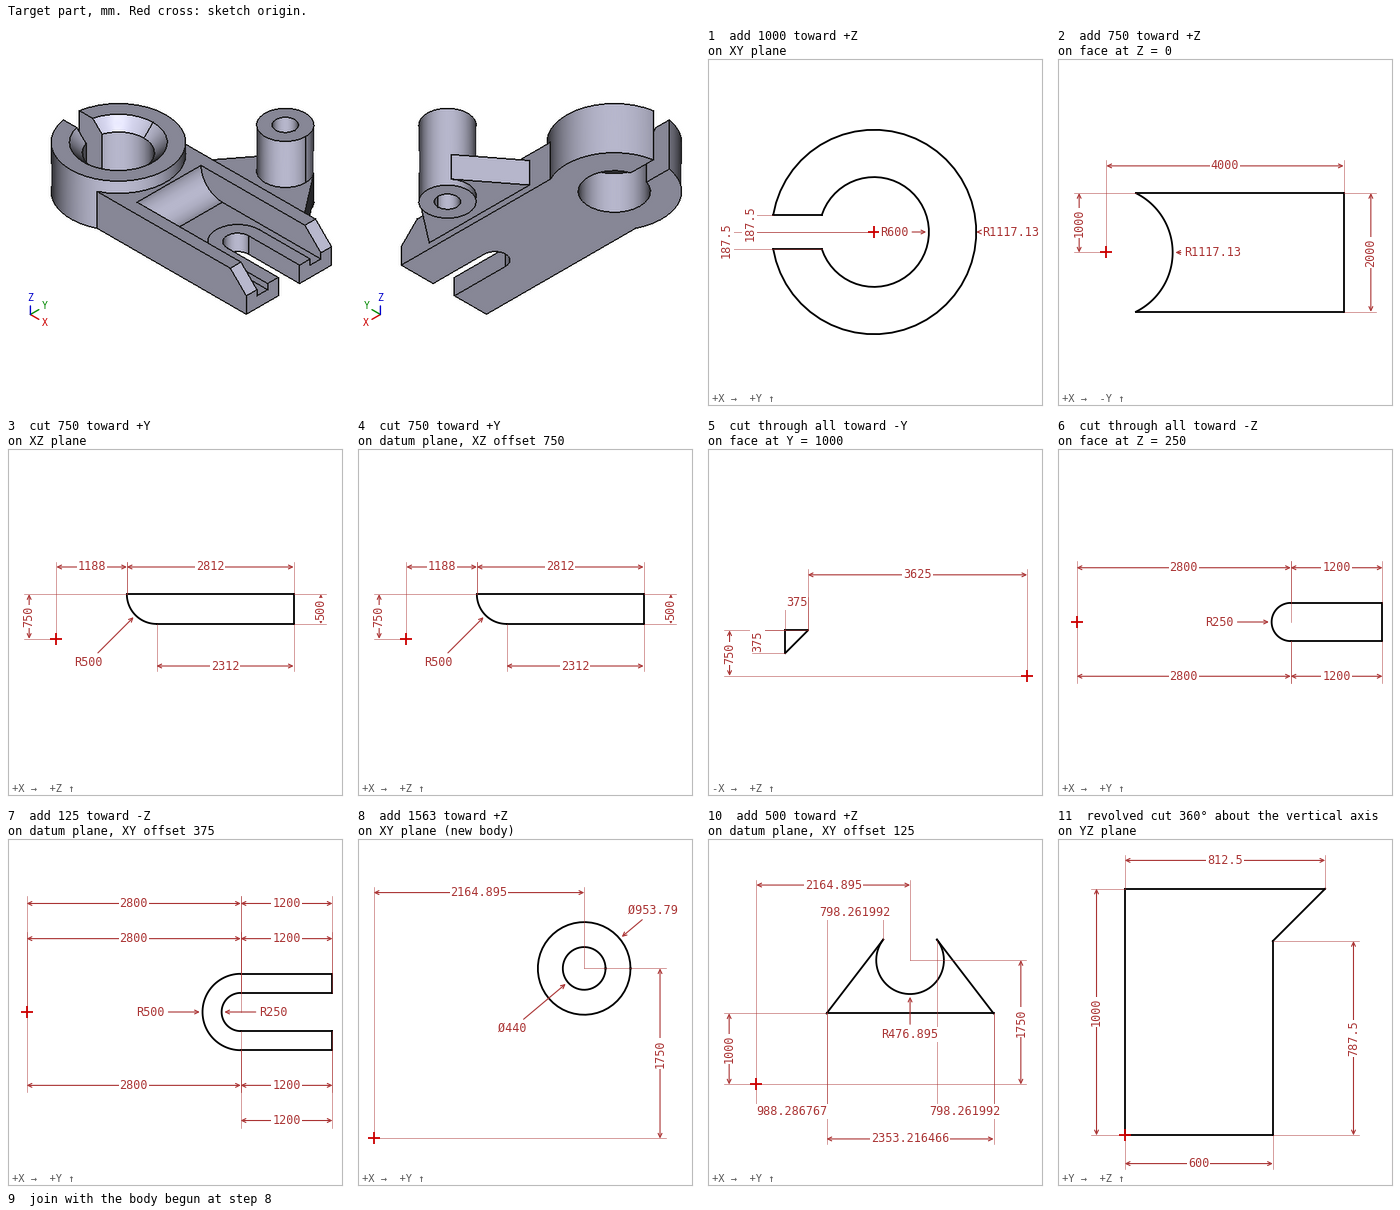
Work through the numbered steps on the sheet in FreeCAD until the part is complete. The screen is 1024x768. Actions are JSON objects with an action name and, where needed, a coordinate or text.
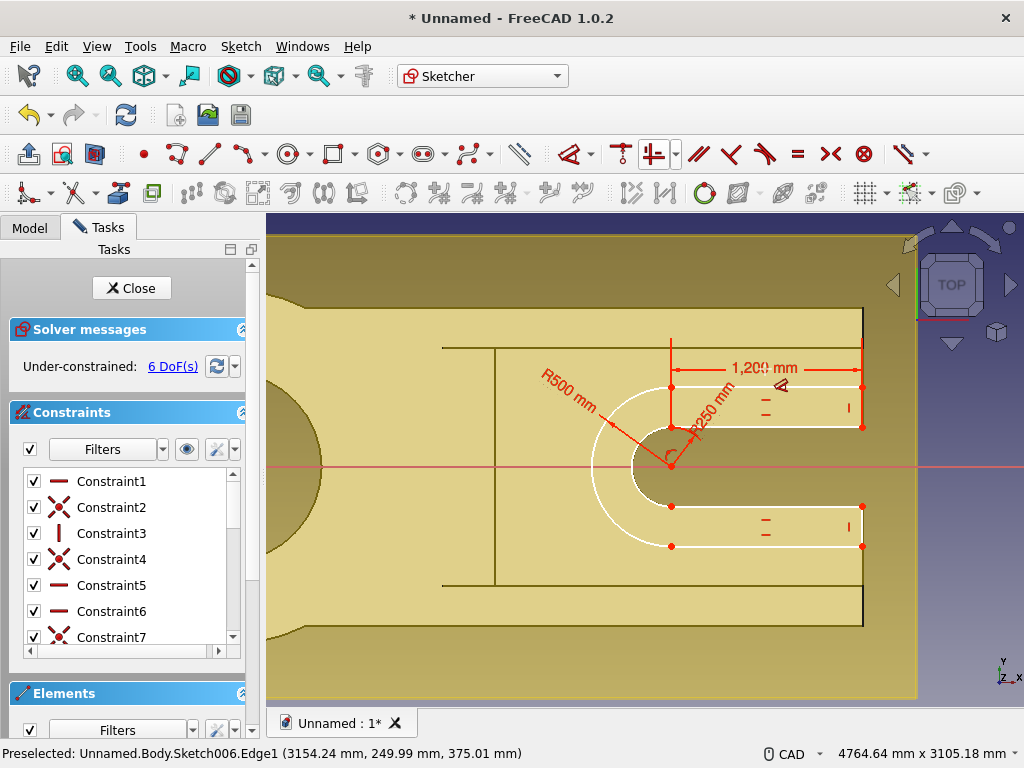
{"action": "left_click", "coordinate": [805, 387]}
{"action": "left_click", "coordinate": [765, 329]}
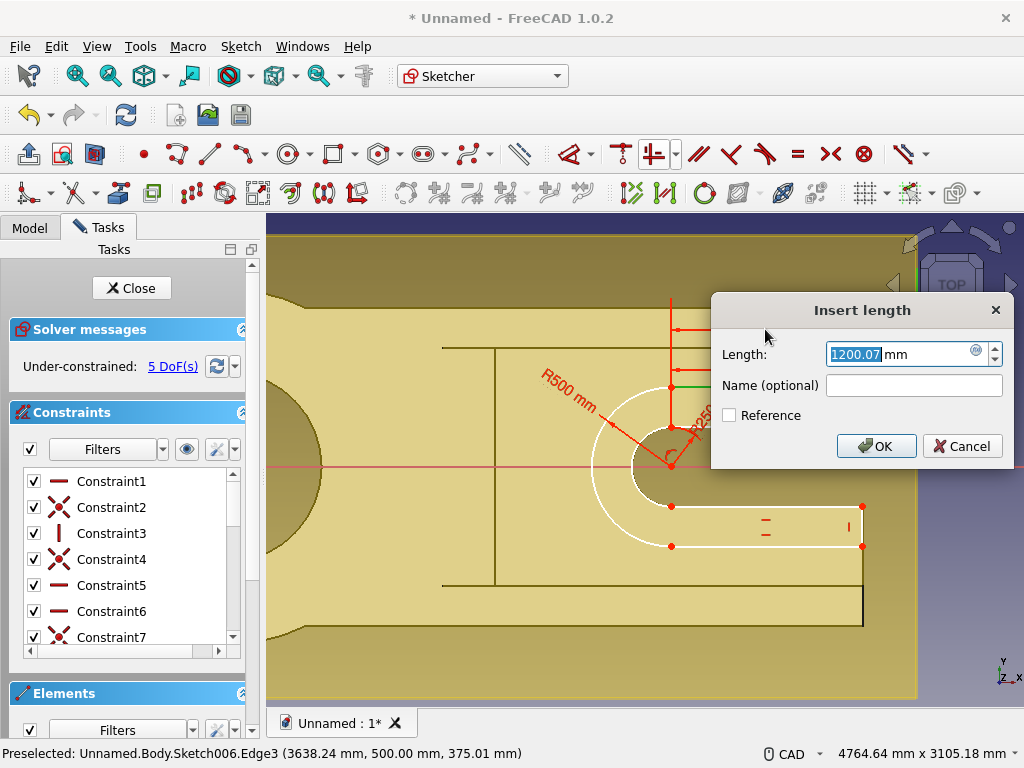
{"action": "type", "text": "1200"}
{"action": "key", "text": "Return"}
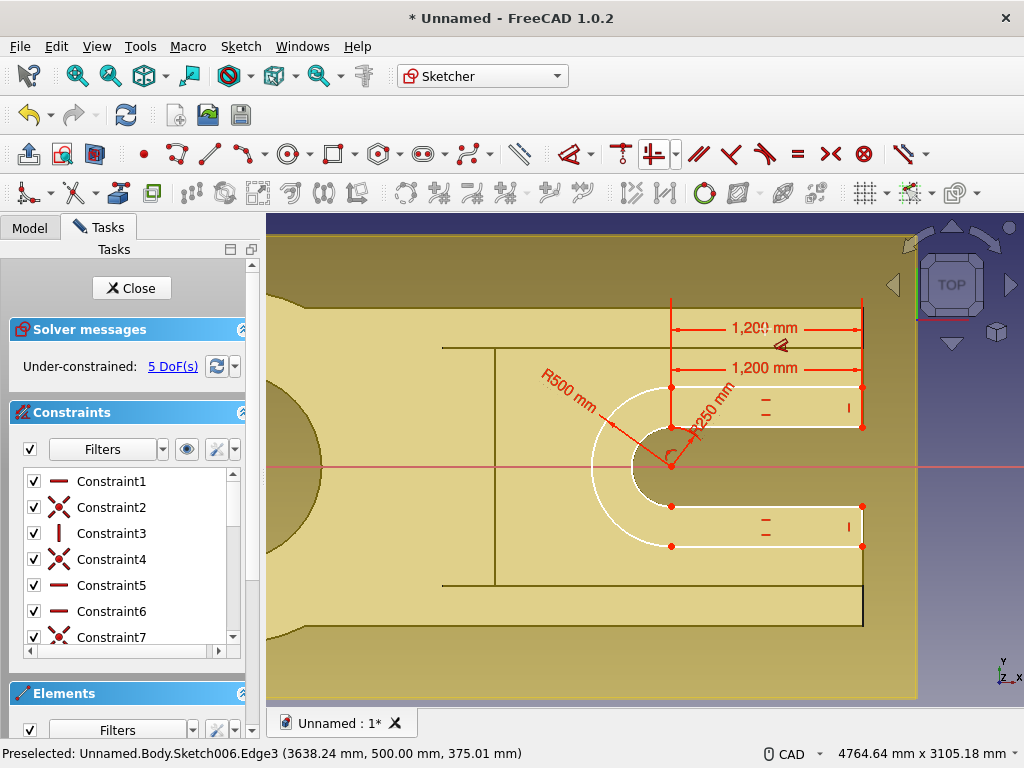
{"action": "left_click", "coordinate": [728, 547]}
{"action": "left_click", "coordinate": [765, 581]}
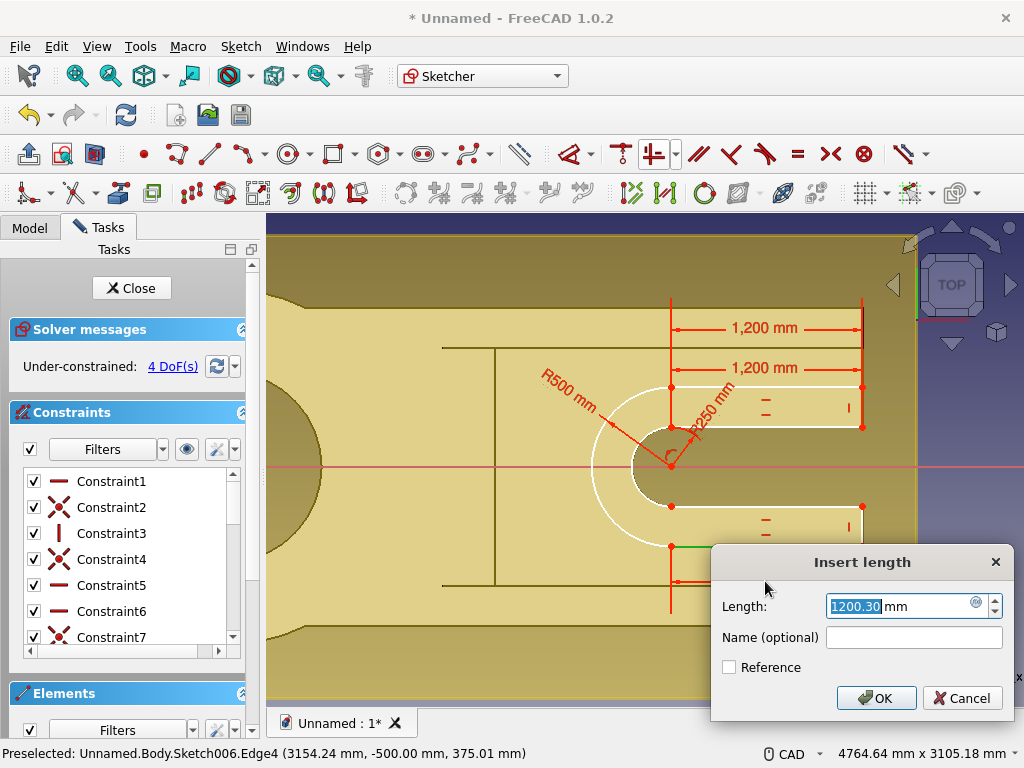
{"action": "type", "text": "1200"}
{"action": "key", "text": "Return"}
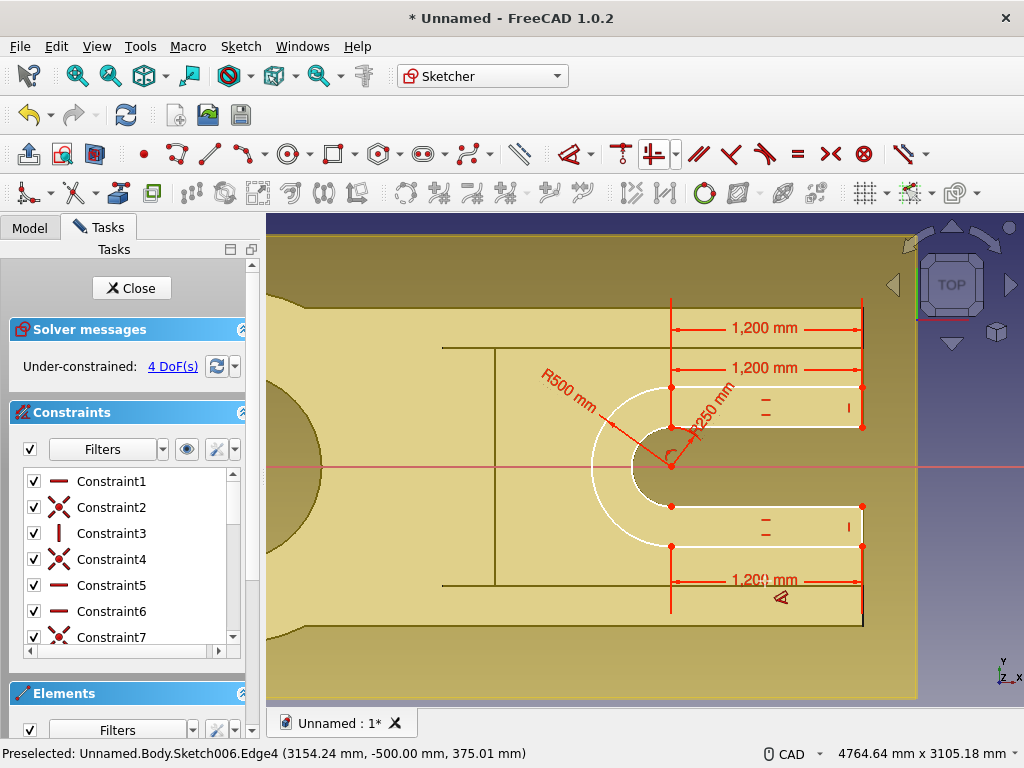
{"action": "left_click", "coordinate": [805, 507]}
{"action": "left_click", "coordinate": [765, 449]}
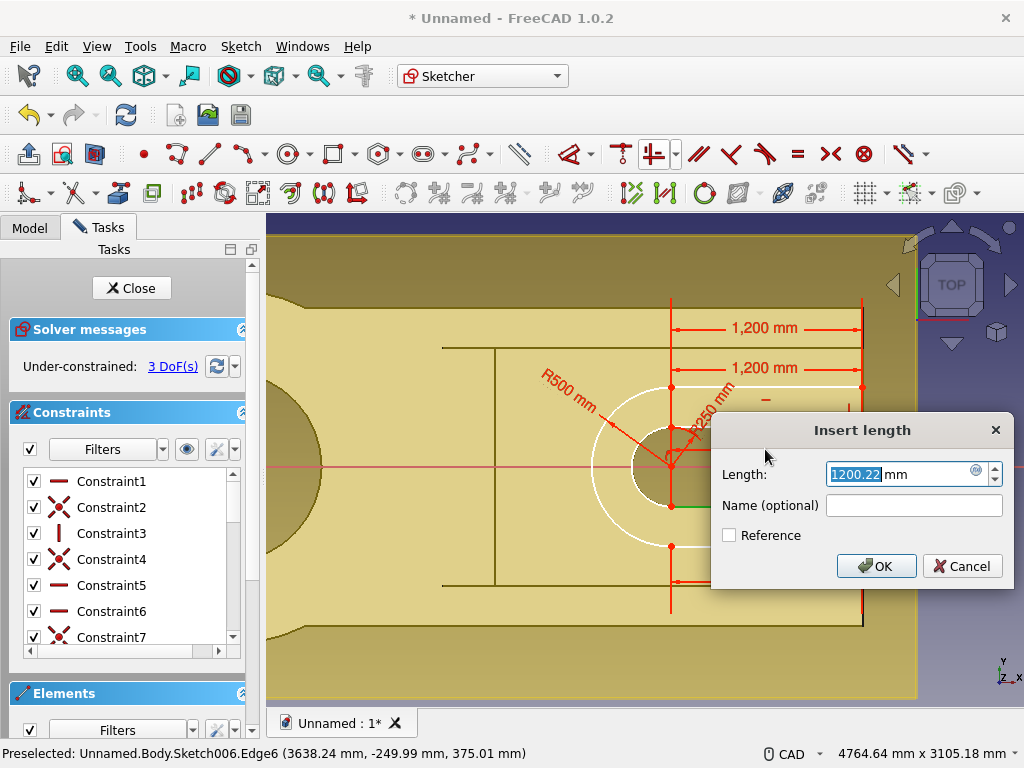
{"action": "type", "text": "1200"}
{"action": "key", "text": "Return"}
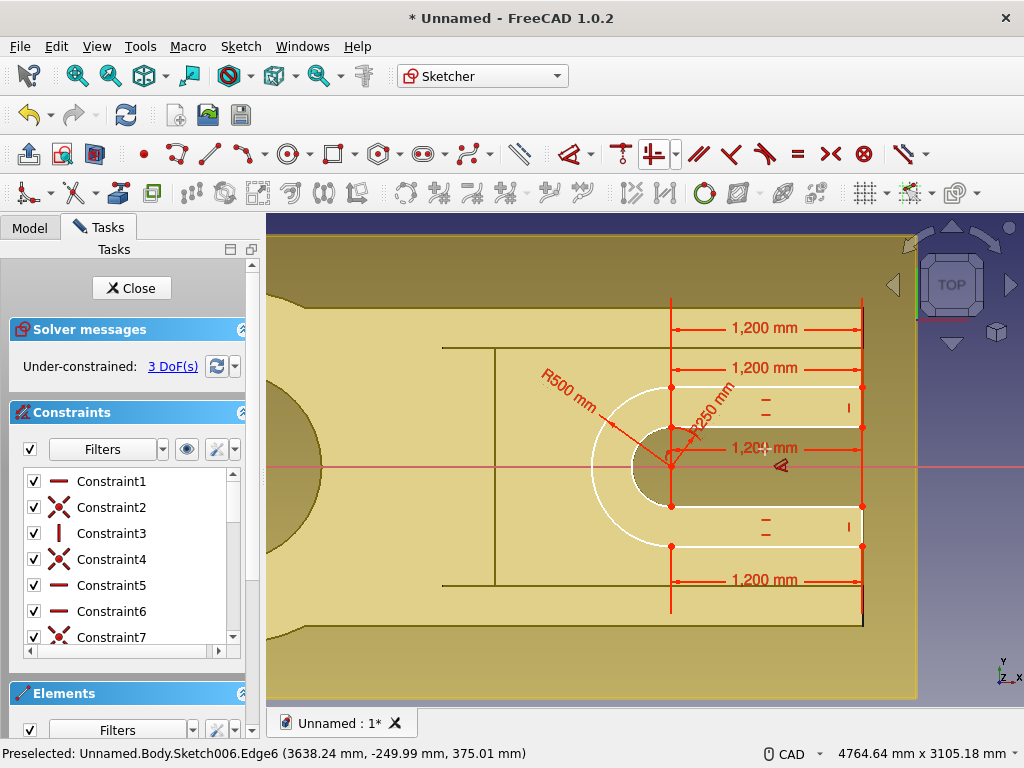
{"action": "left_click", "coordinate": [671, 427]}
{"action": "left_click", "coordinate": [483, 393]}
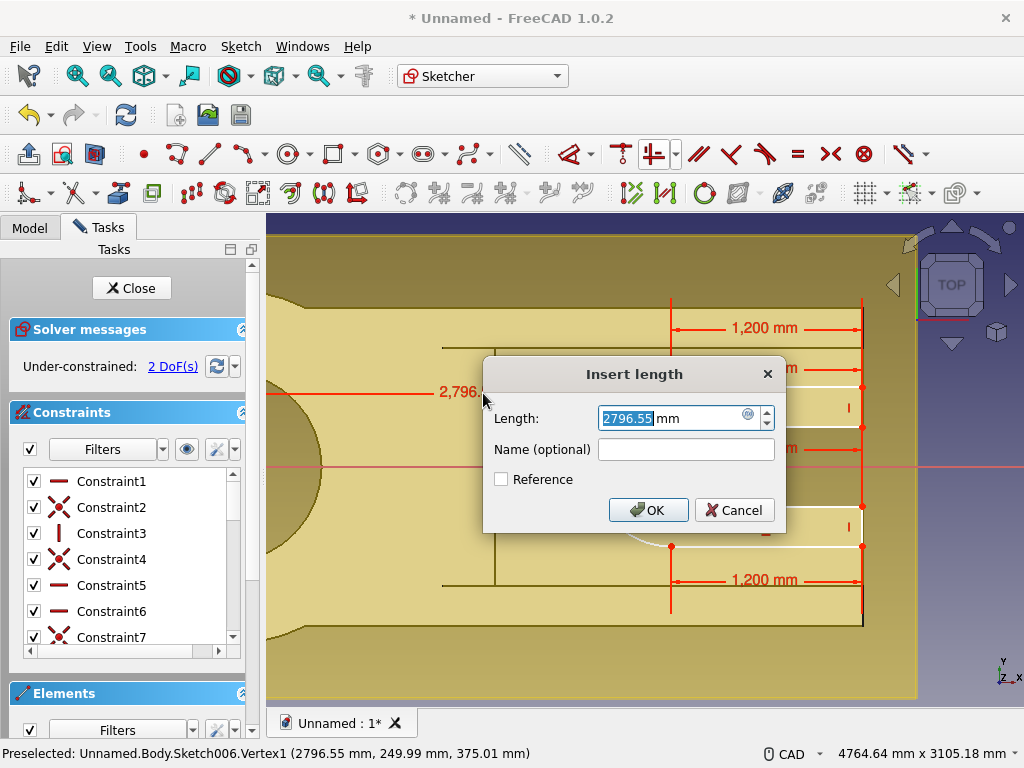
{"action": "type", "text": "2800"}
{"action": "key", "text": "Return"}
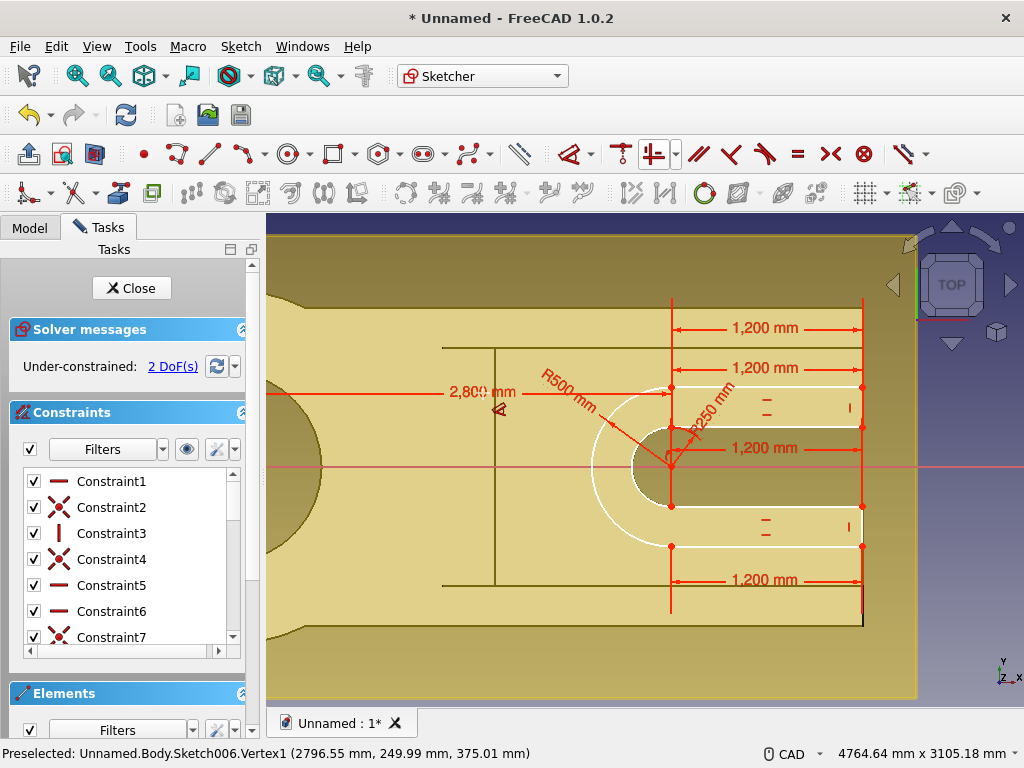
{"action": "left_click", "coordinate": [671, 547]}
{"action": "left_click", "coordinate": [483, 581]}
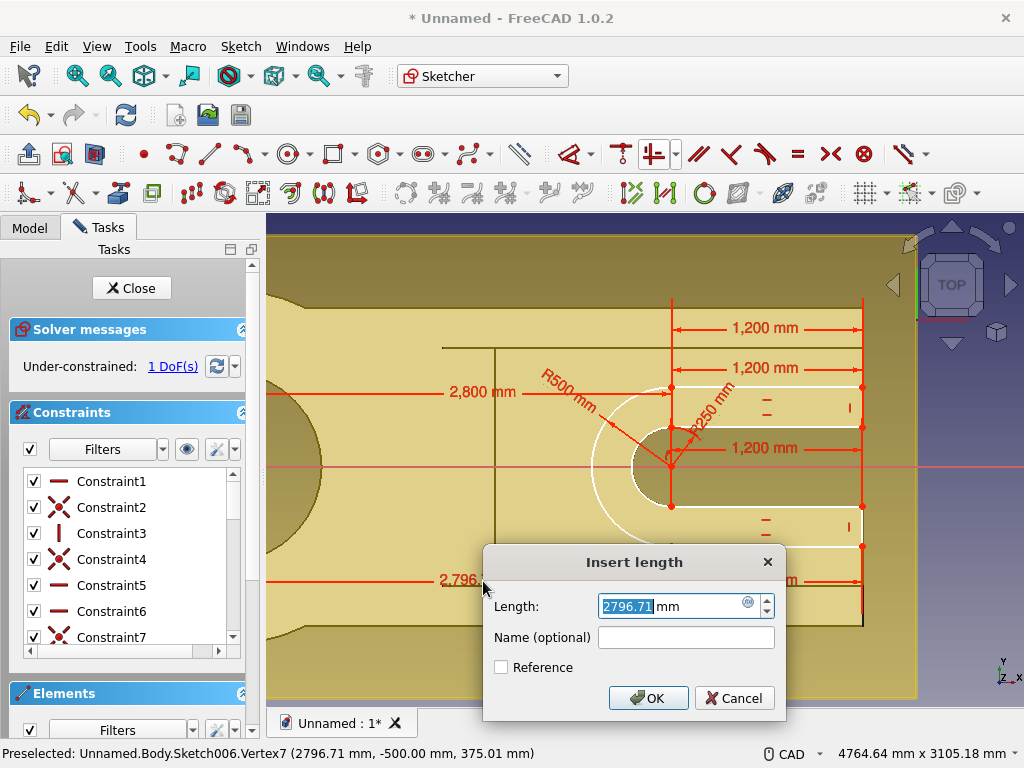
{"action": "type", "text": "2800"}
{"action": "key", "text": "Return"}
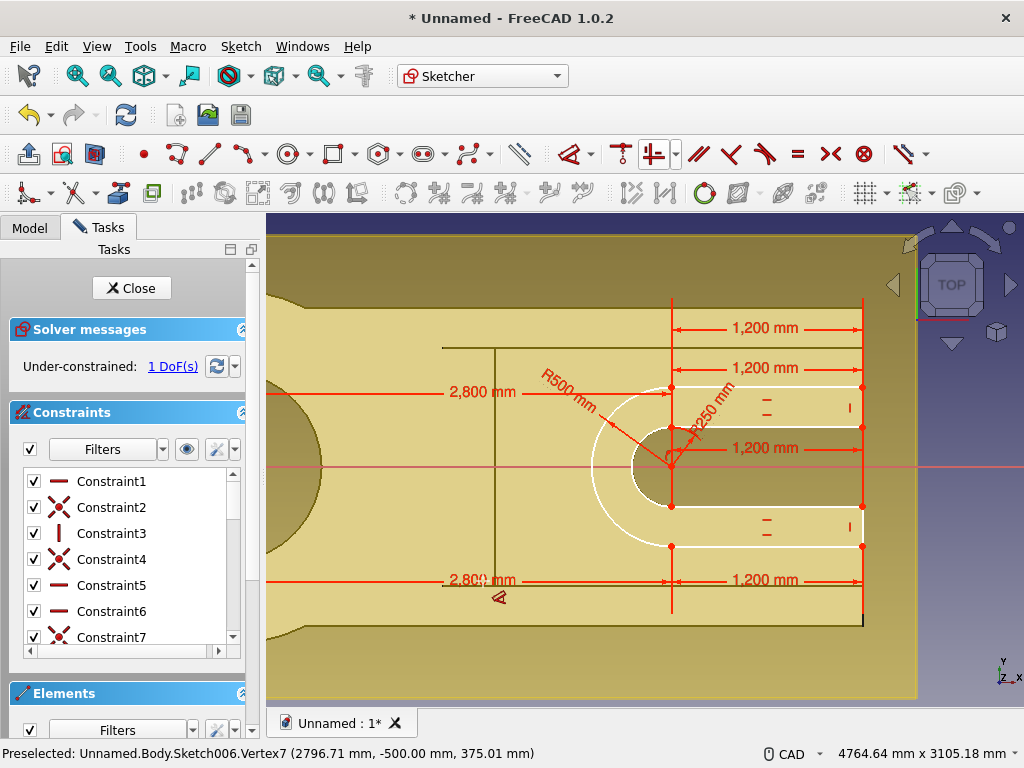
{"action": "left_click", "coordinate": [671, 467]}
{"action": "left_click", "coordinate": [483, 501]}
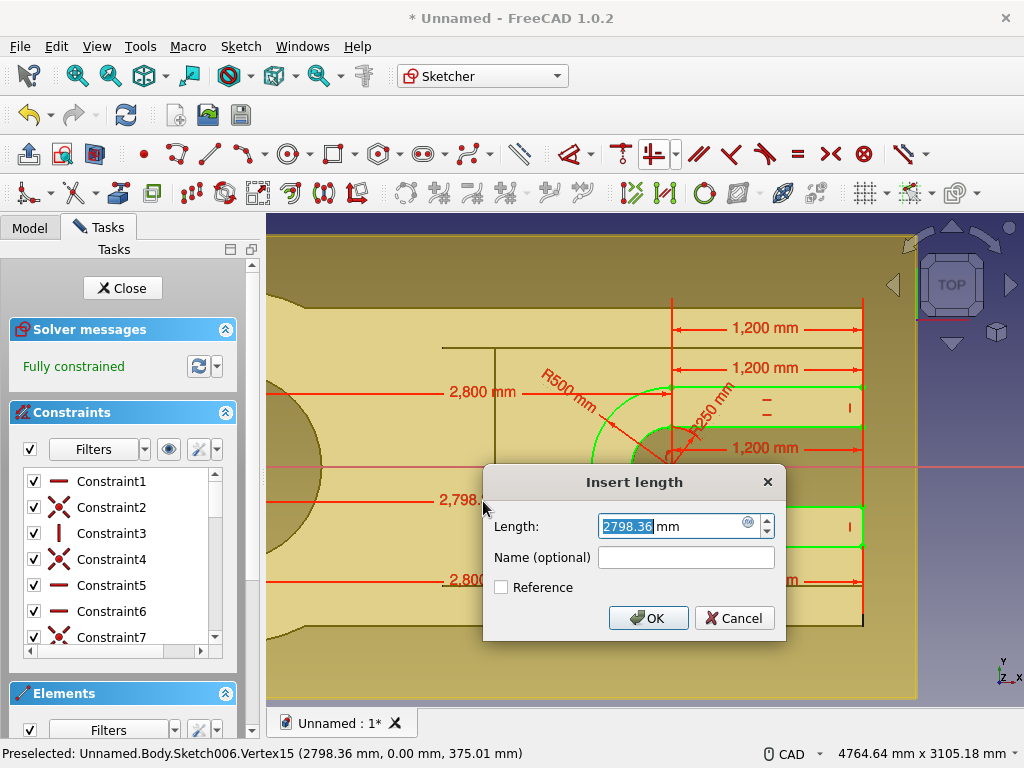
{"action": "type", "text": "2800"}
{"action": "key", "text": "Return"}
{"action": "key", "text": "Escape"}